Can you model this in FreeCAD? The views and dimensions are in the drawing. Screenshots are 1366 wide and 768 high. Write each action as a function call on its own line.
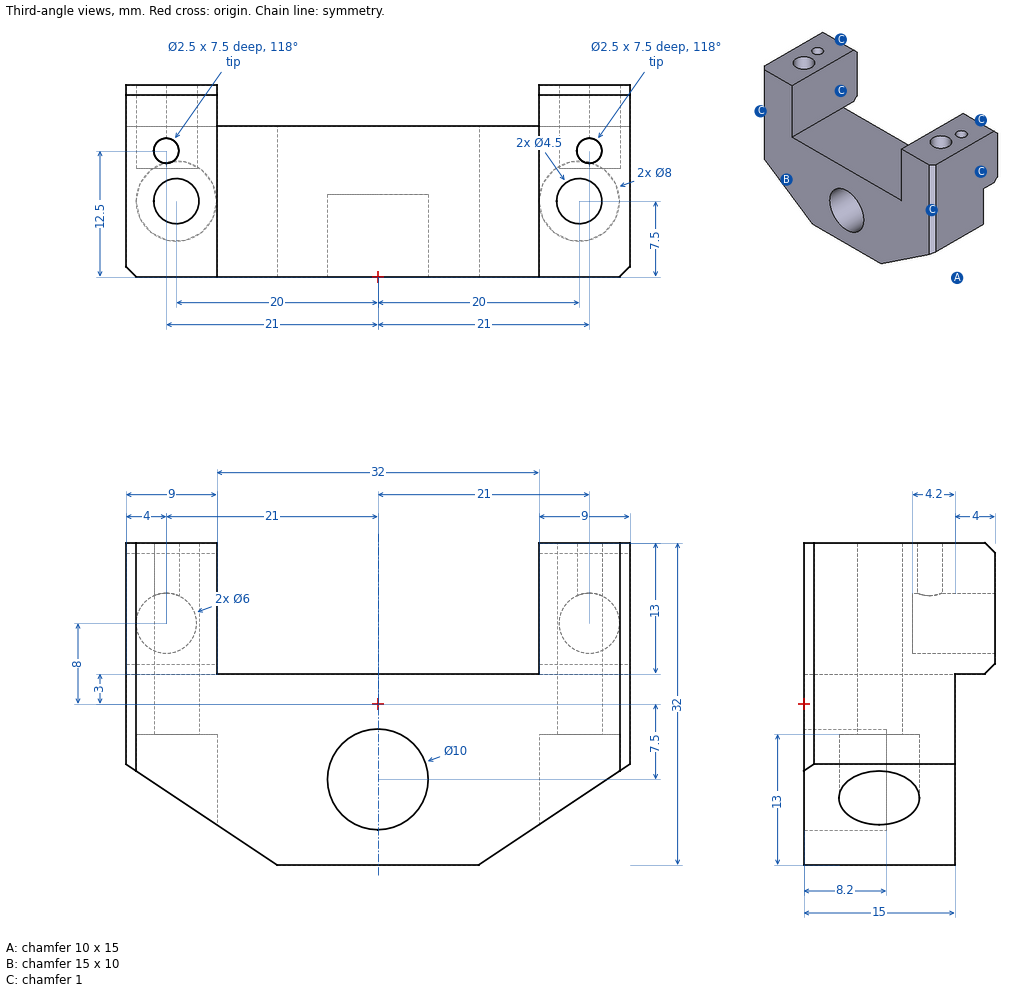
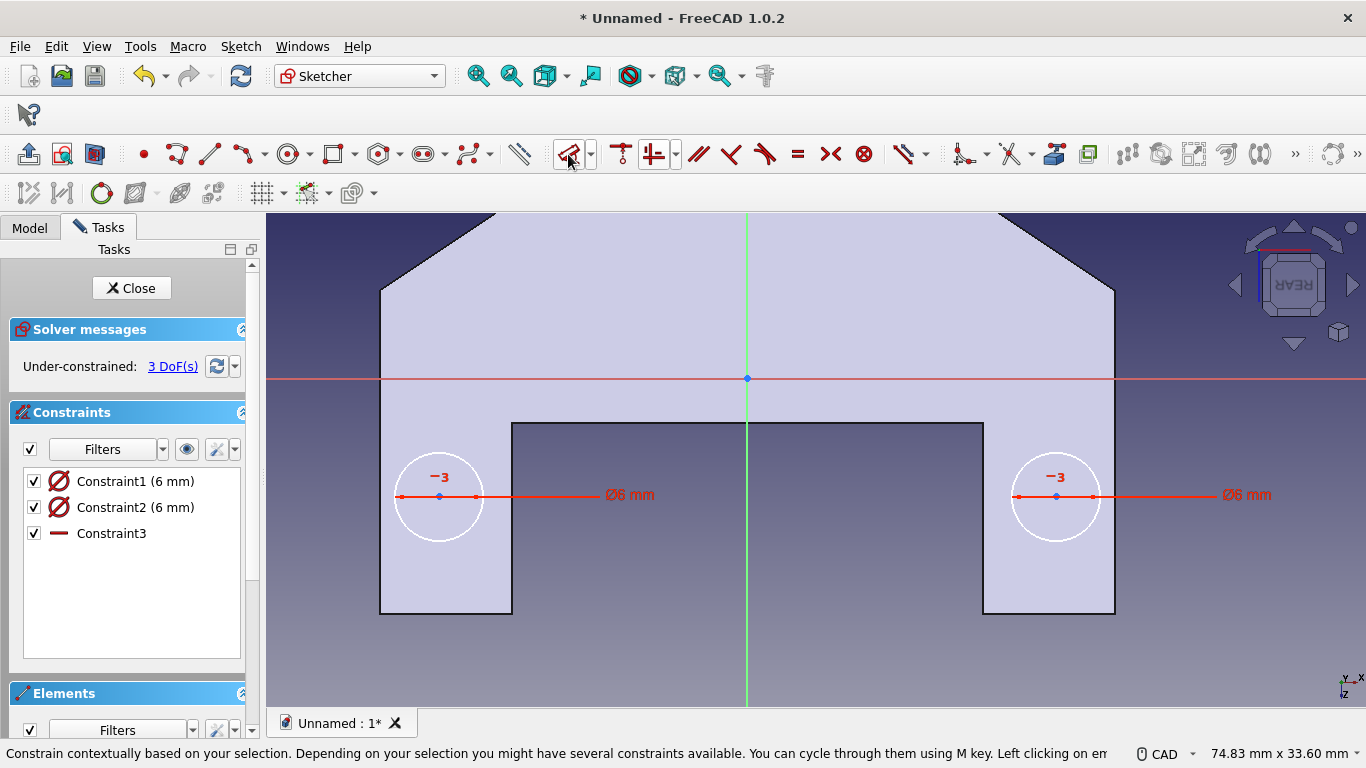
click(439, 497)
click(405, 438)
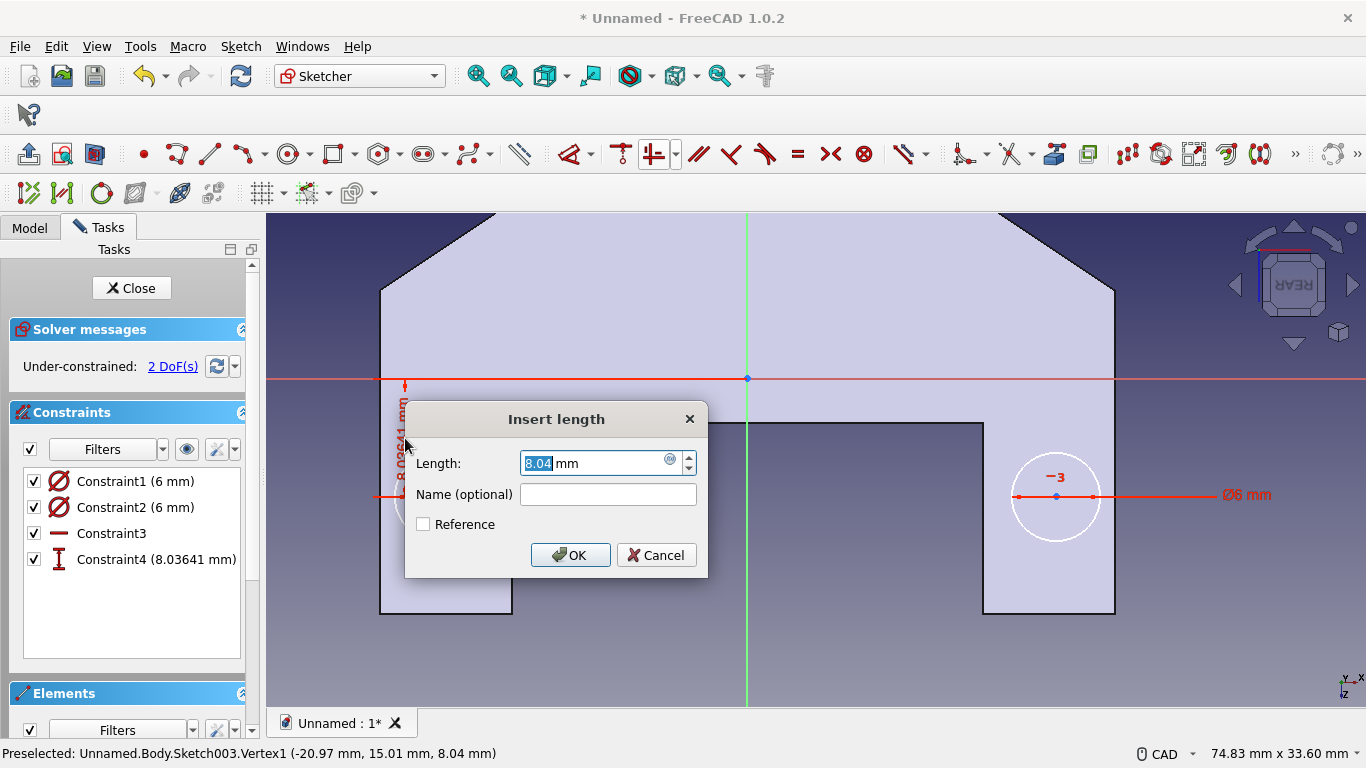
text(8)
key(Return)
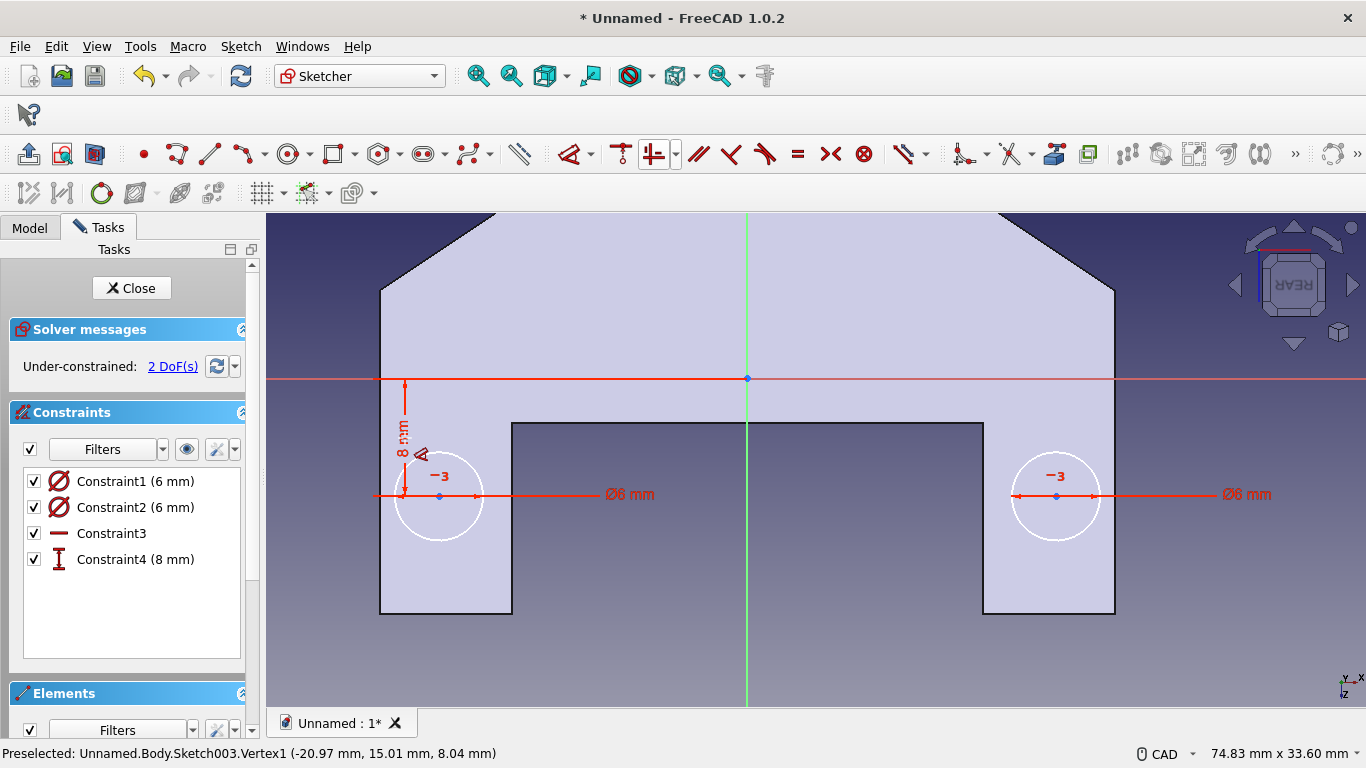
click(439, 496)
click(593, 345)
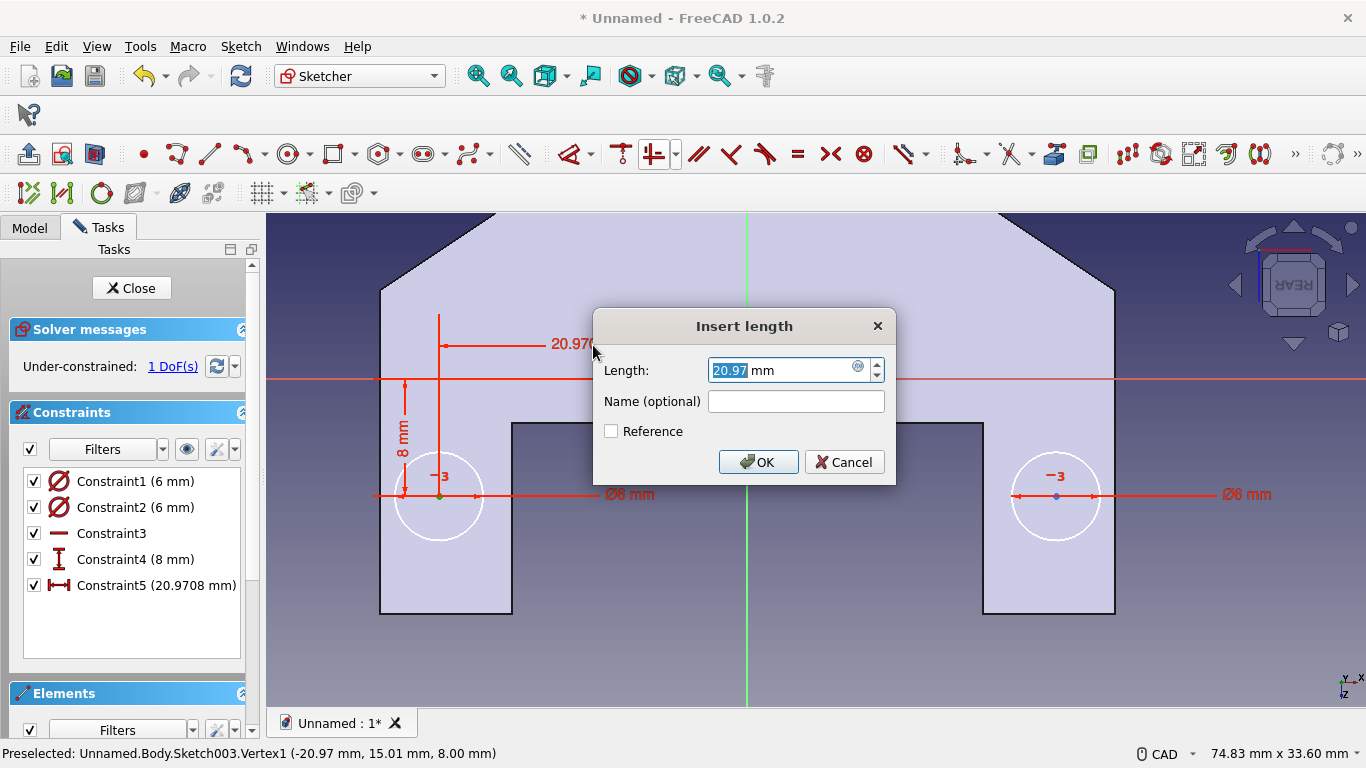
text(21)
key(Return)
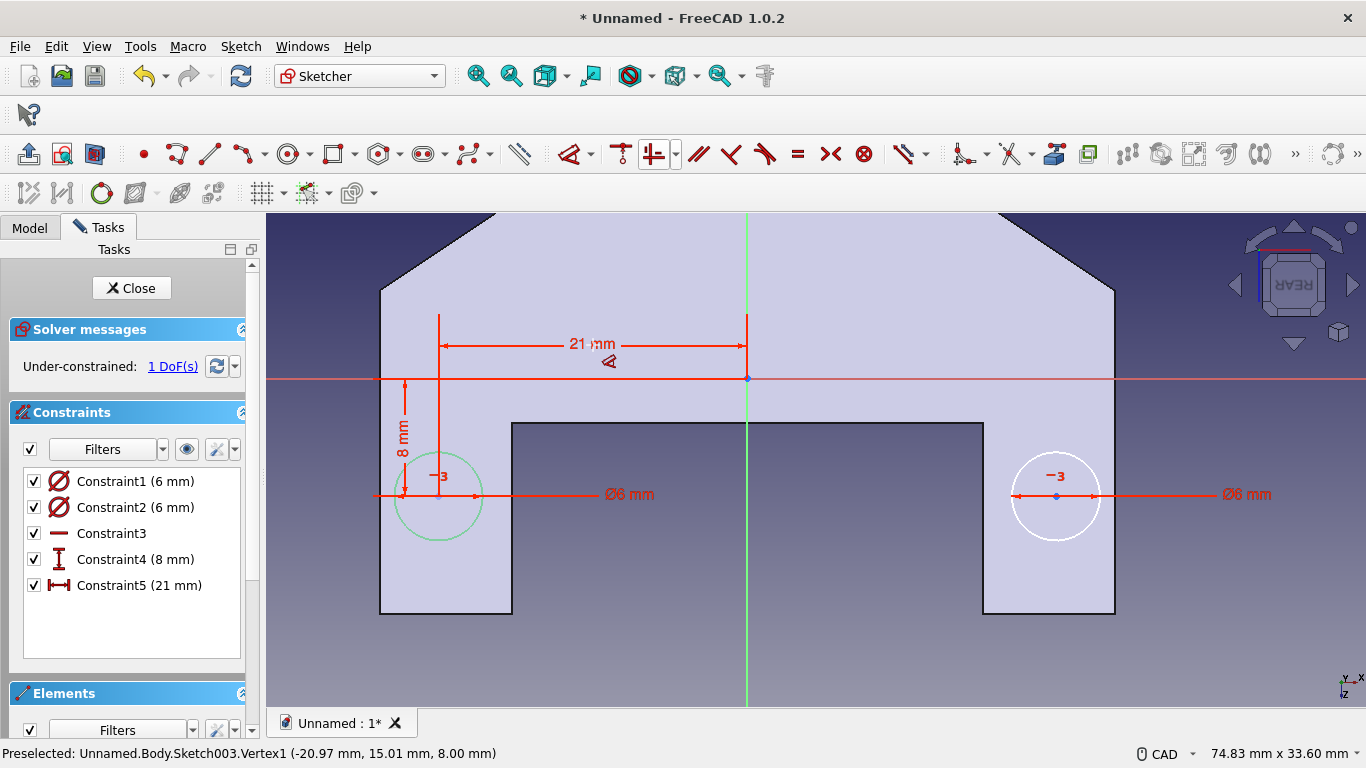
click(1056, 496)
click(902, 345)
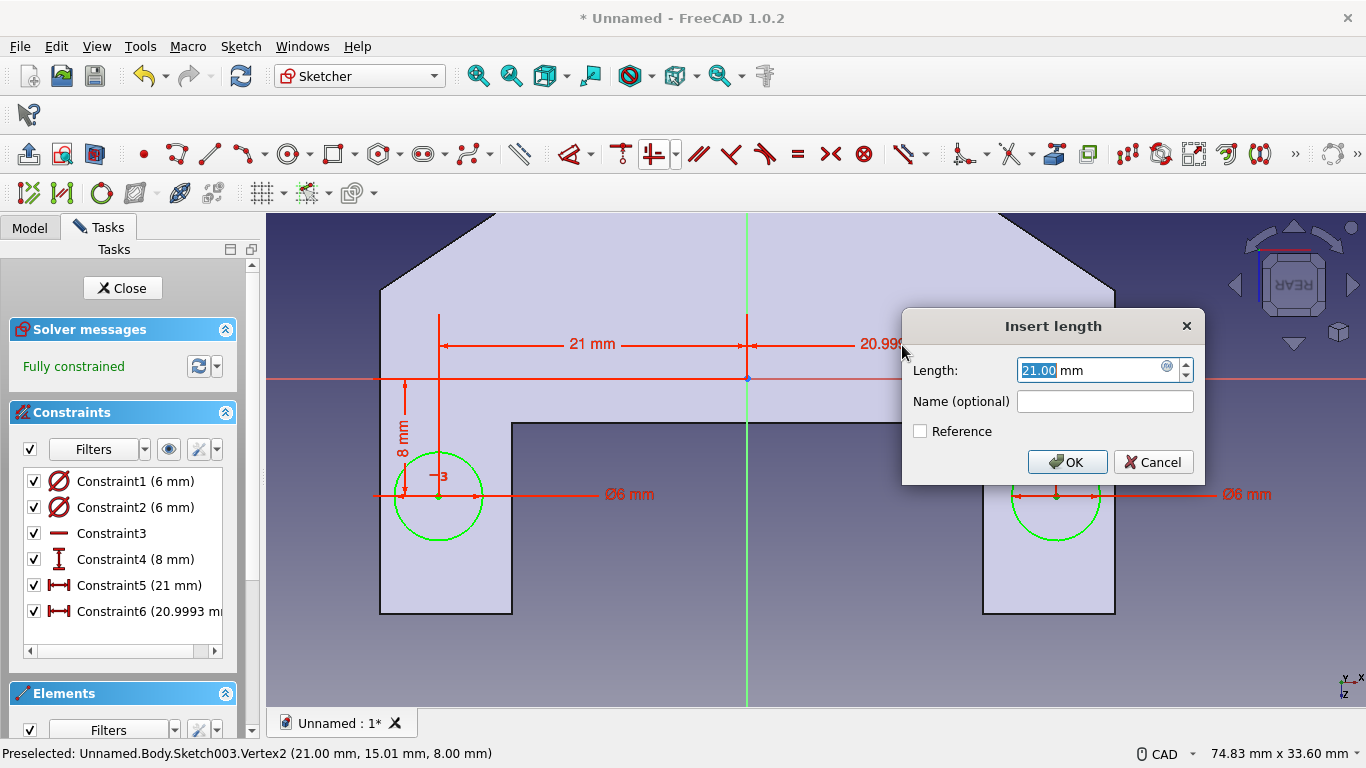
text(21)
key(Return)
key(Escape)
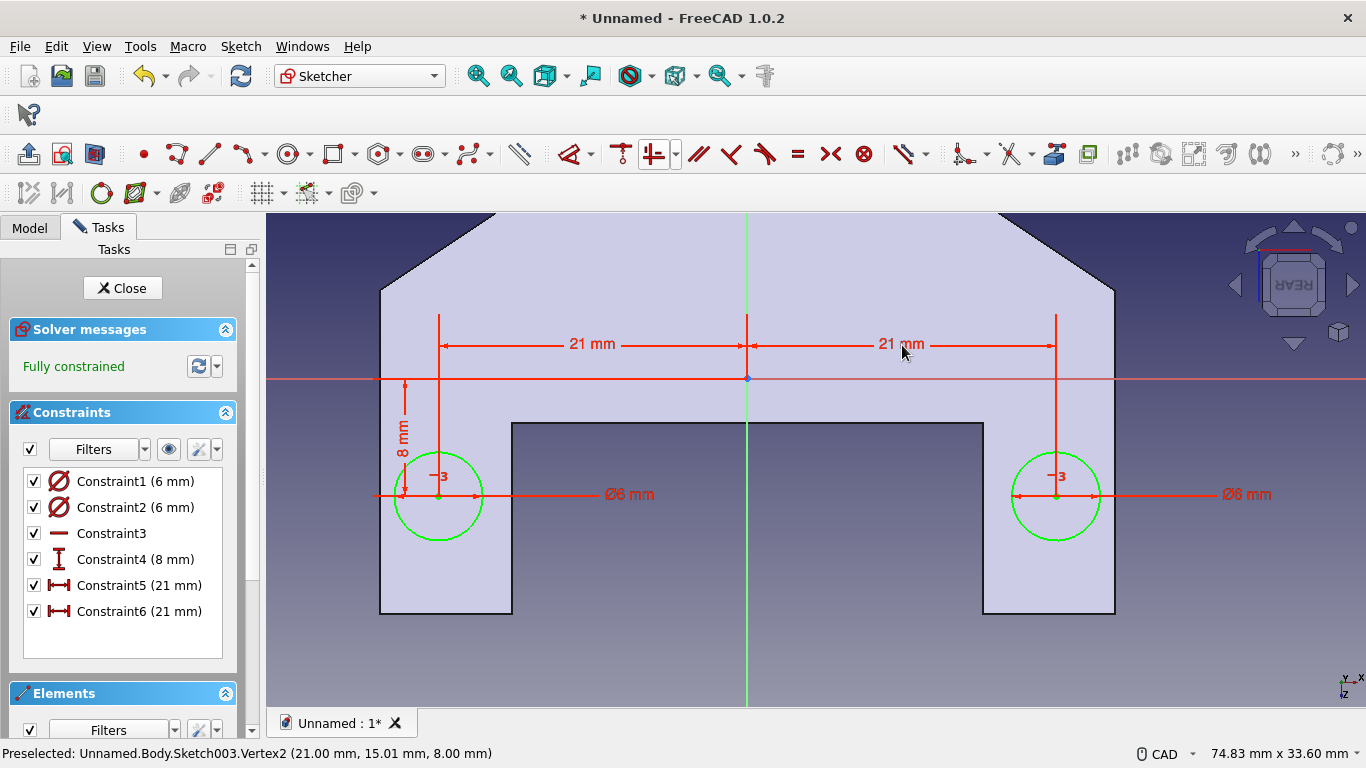
click(123, 288)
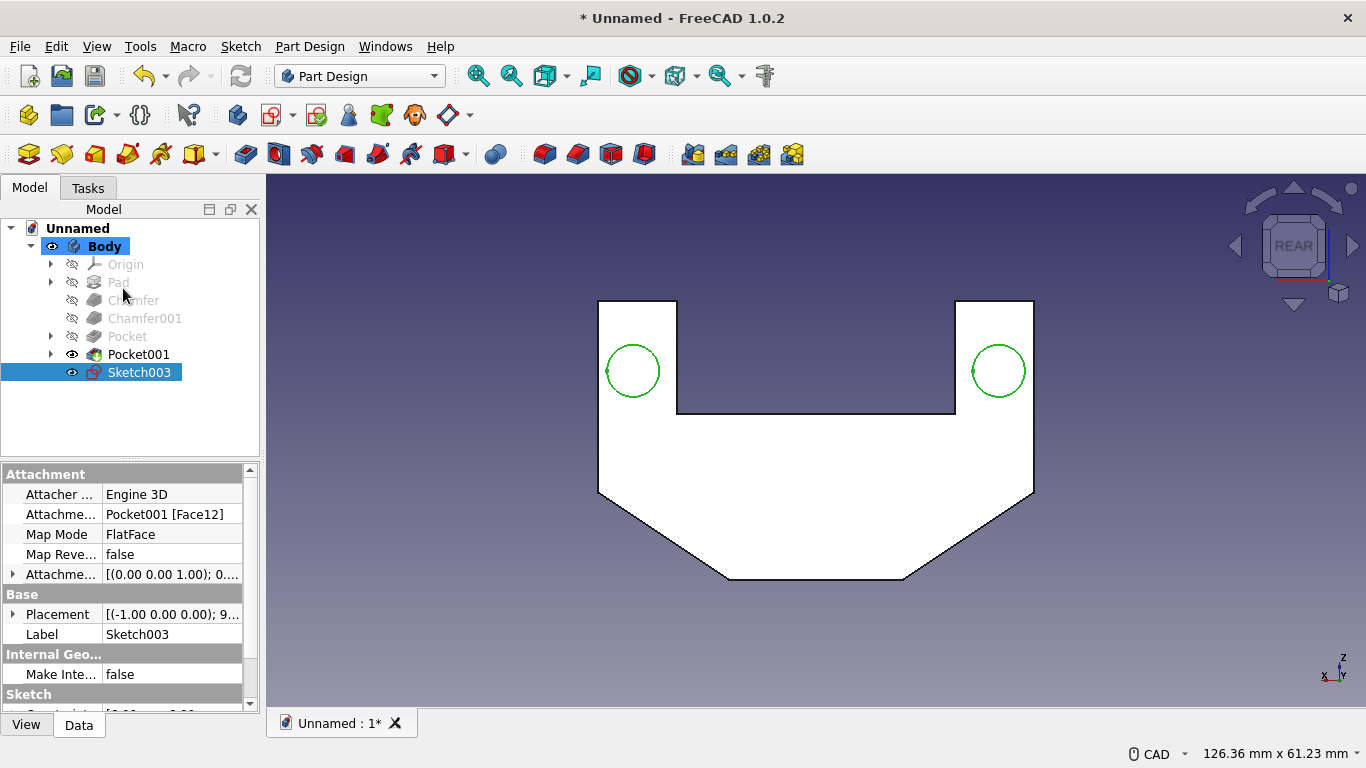
click(246, 154)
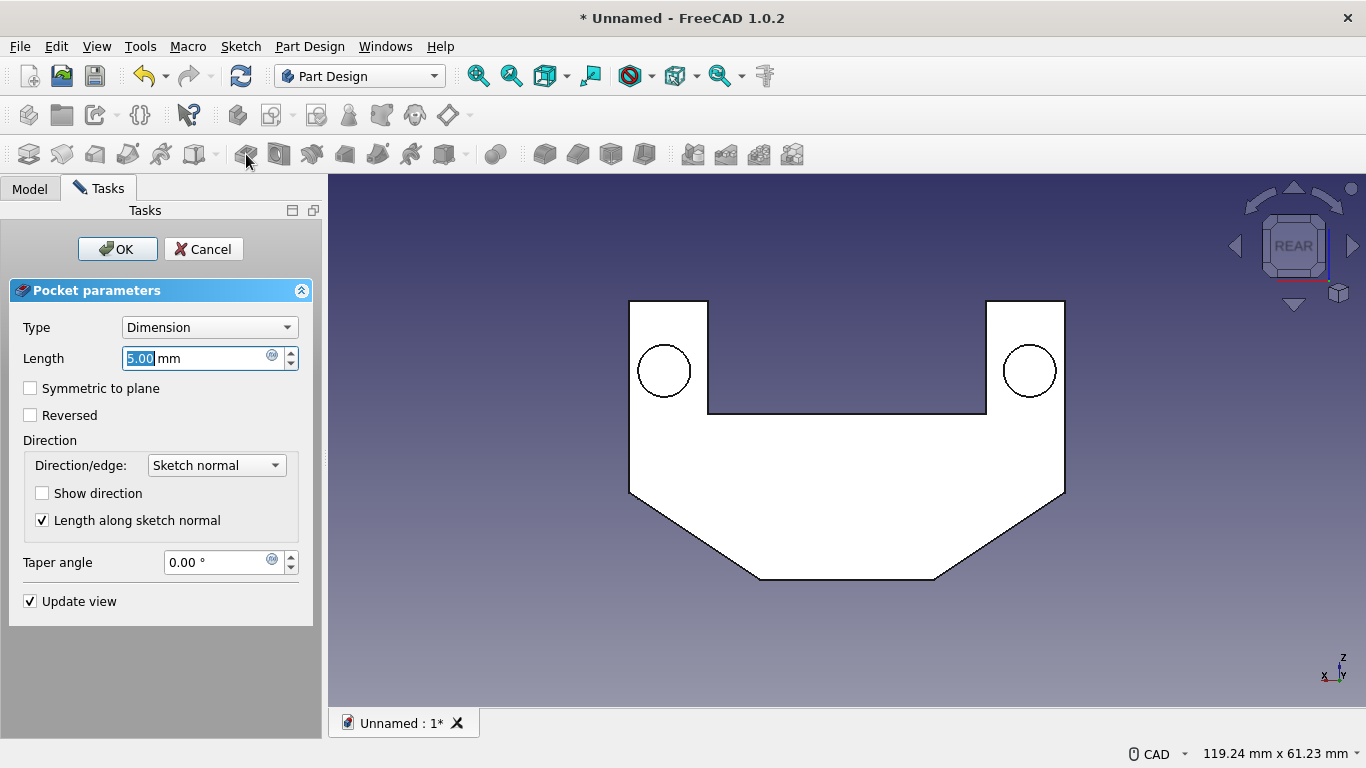
text(4.2)
key(Tab)